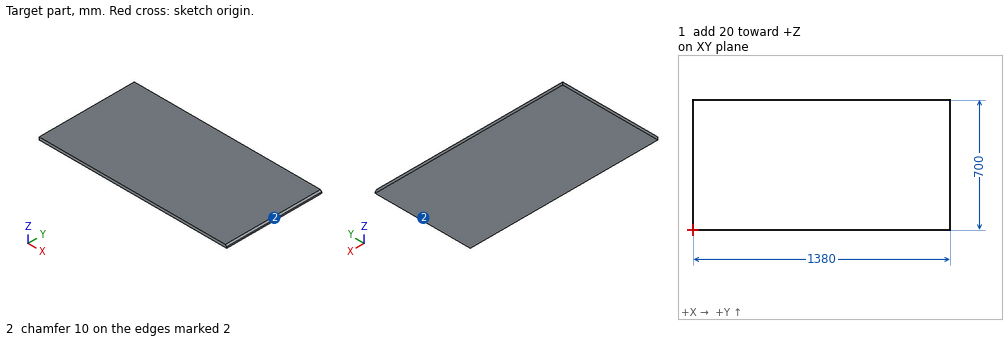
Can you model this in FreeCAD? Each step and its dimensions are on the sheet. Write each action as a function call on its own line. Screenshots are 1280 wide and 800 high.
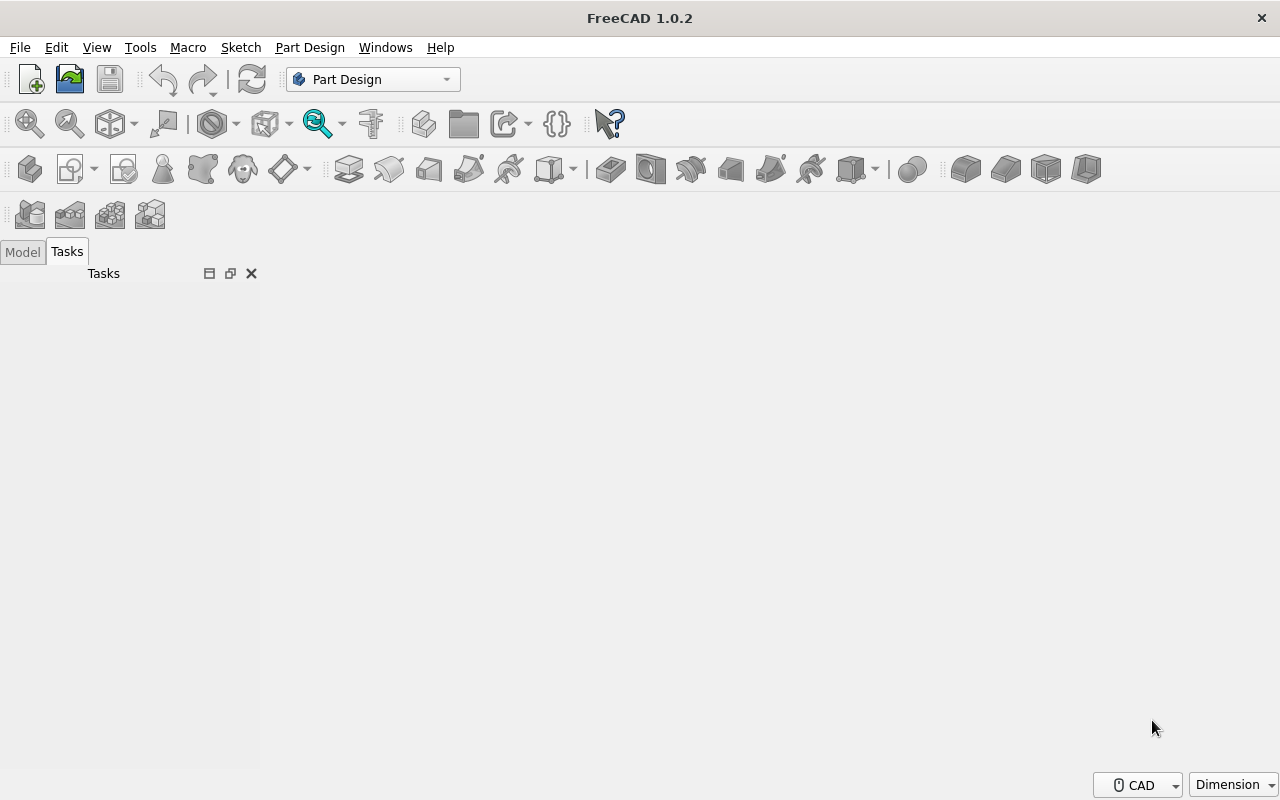
click(30, 80)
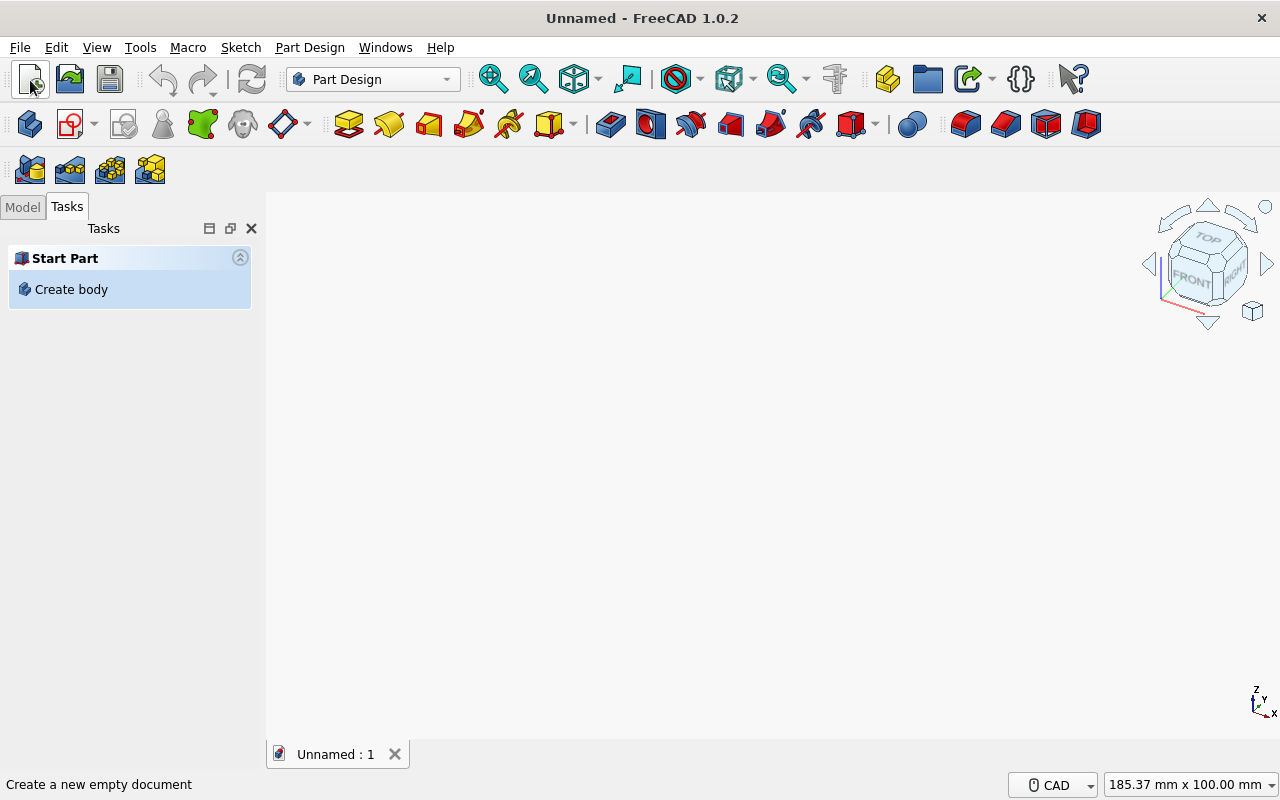
click(70, 124)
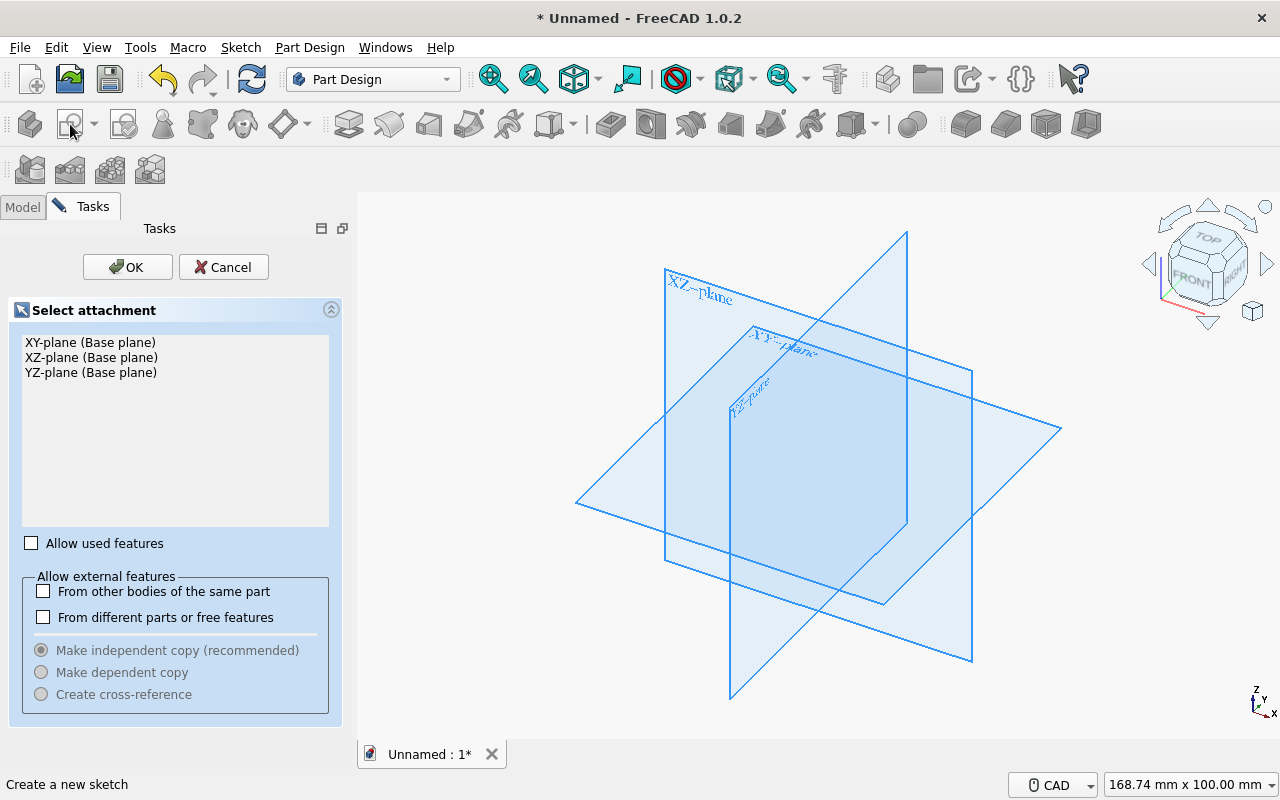
click(82, 342)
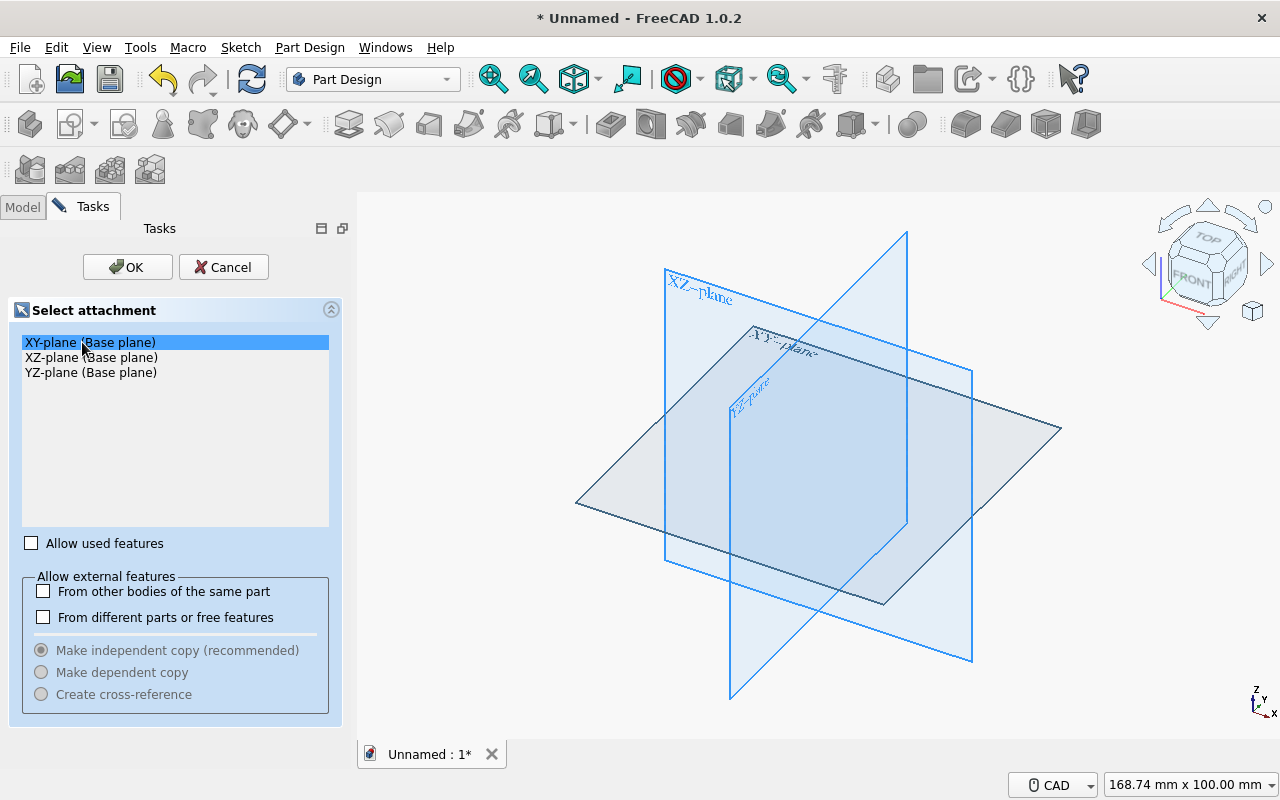
click(128, 267)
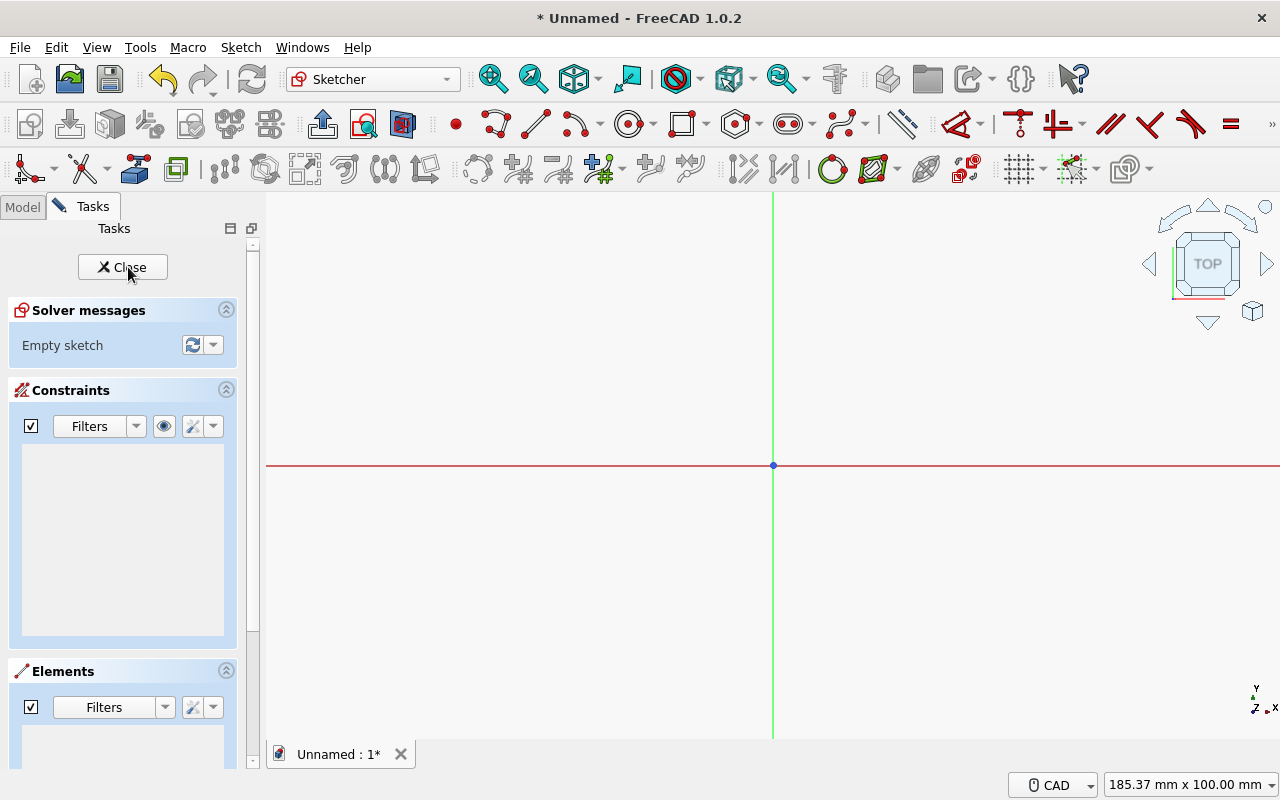
scroll(396, 619, down, 13)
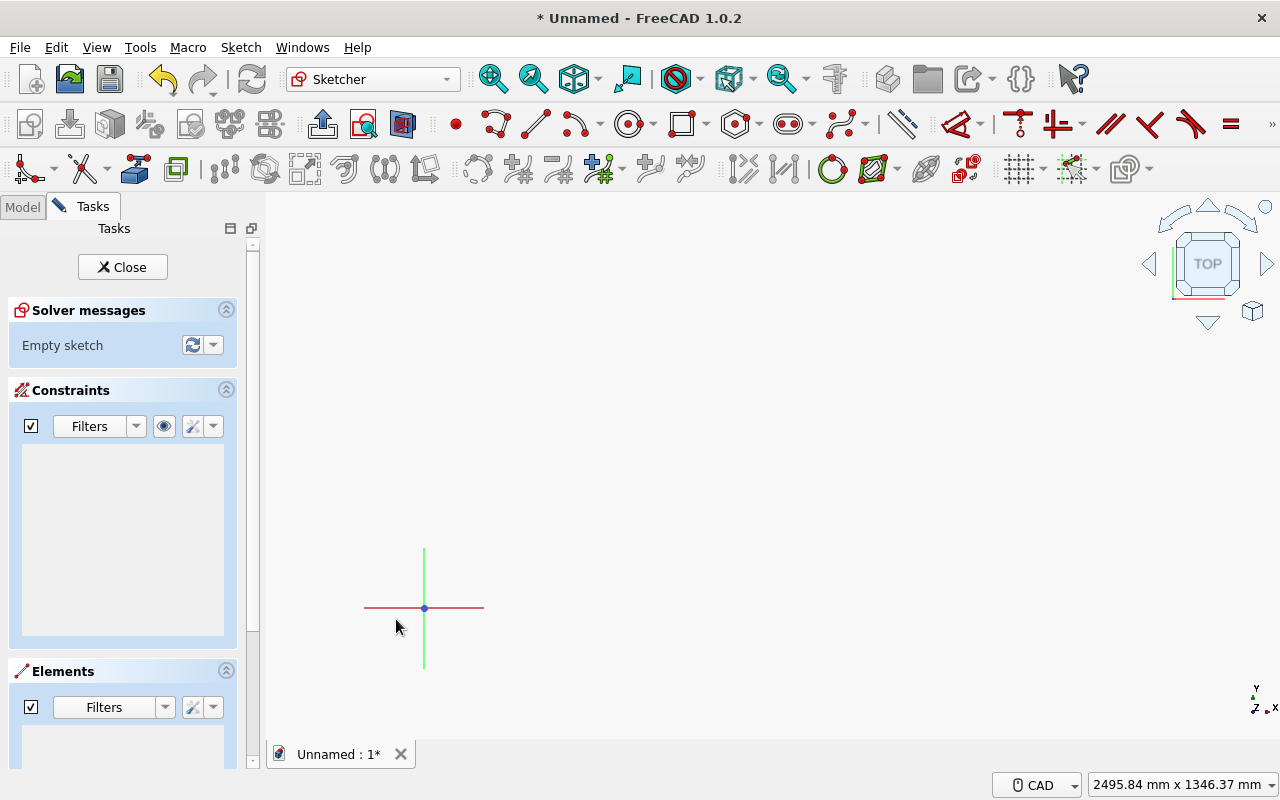
click(682, 124)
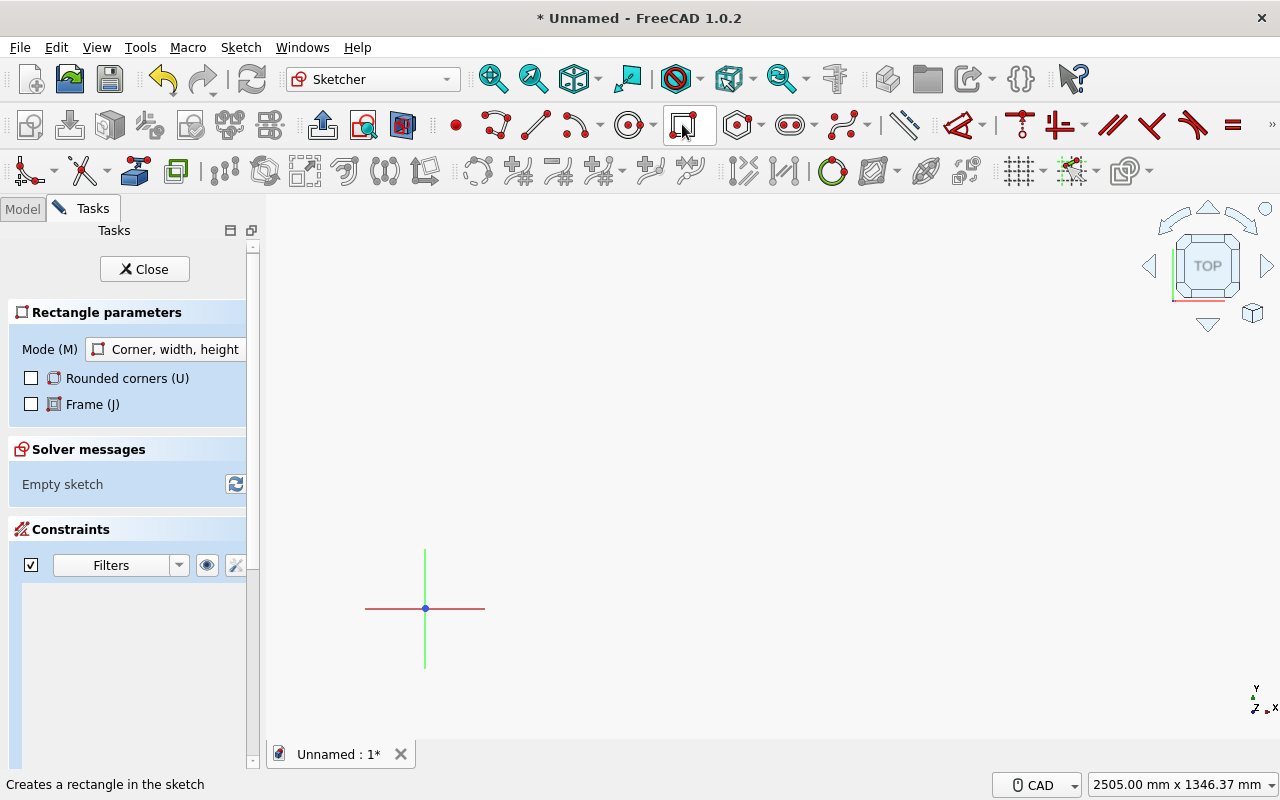
click(425, 609)
move(984, 325)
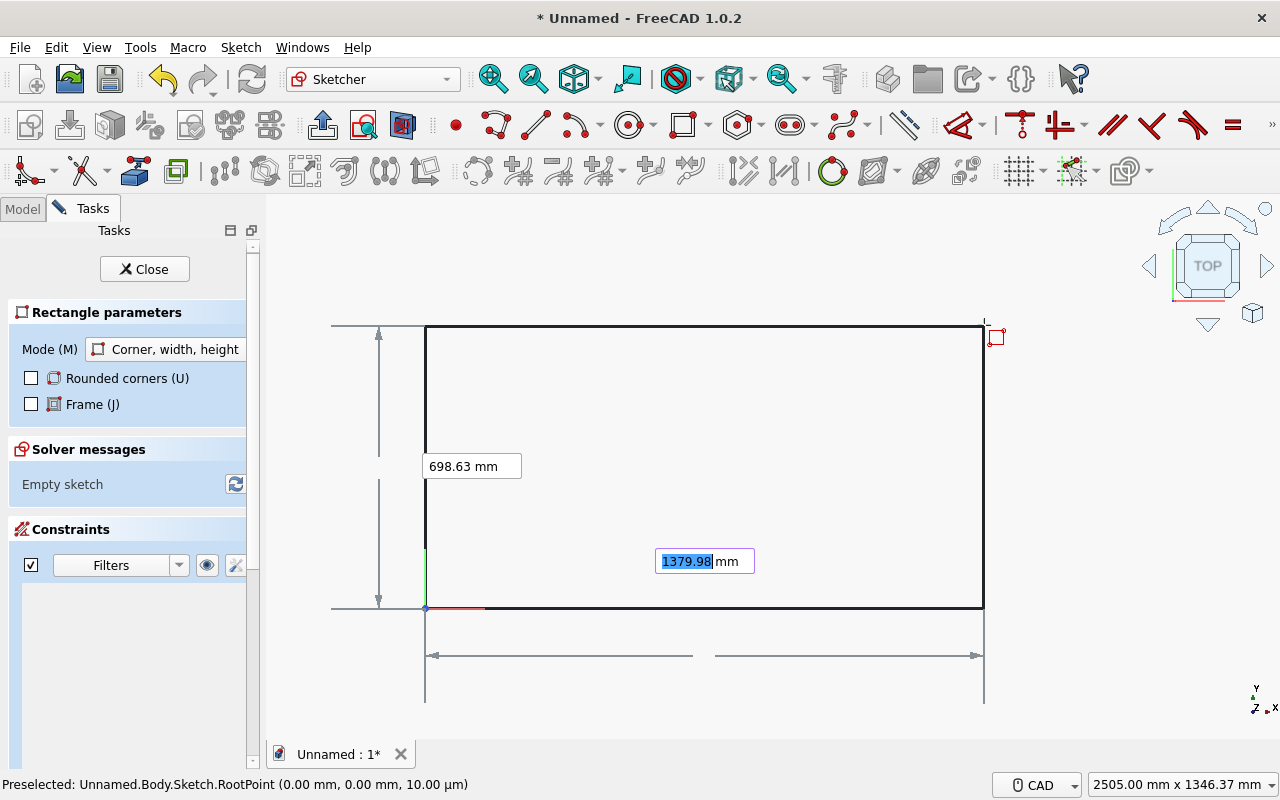
text(1380)
key(Tab)
text(700)
key(Return)
key(Escape)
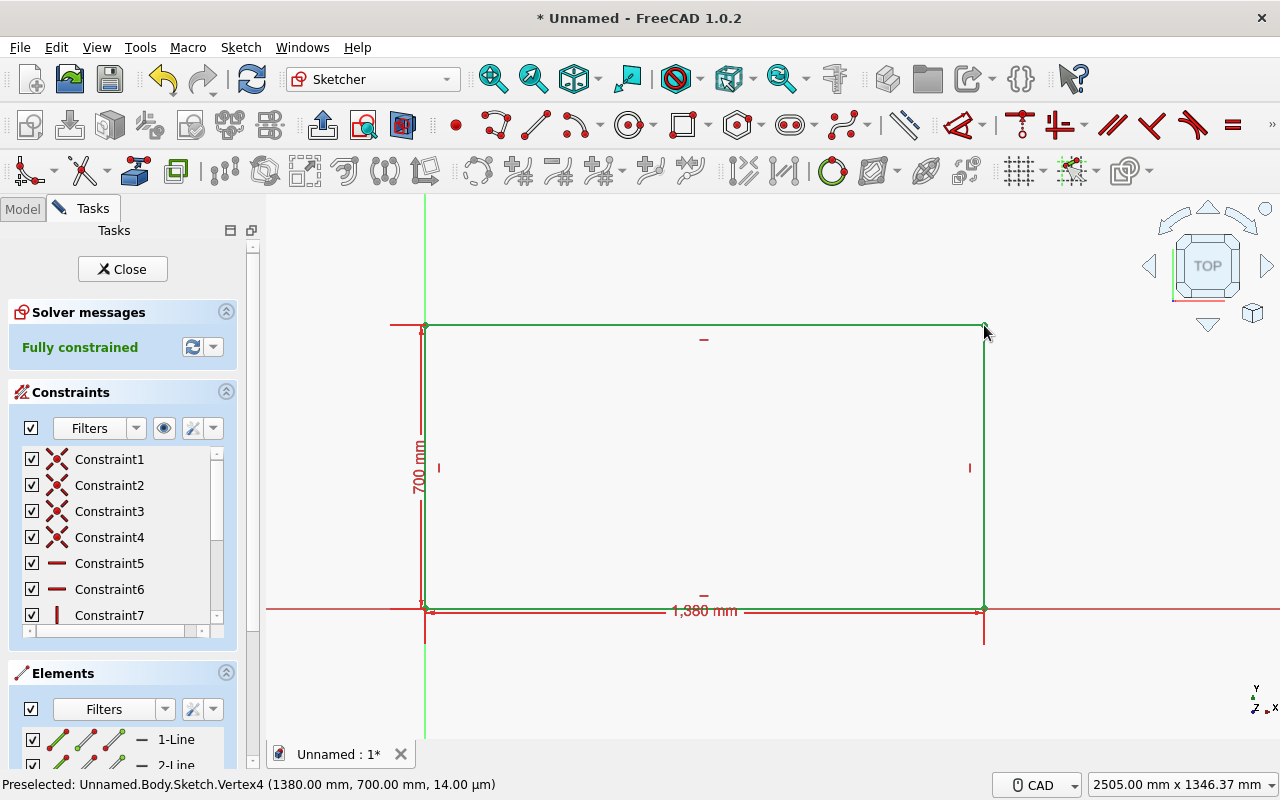
click(123, 269)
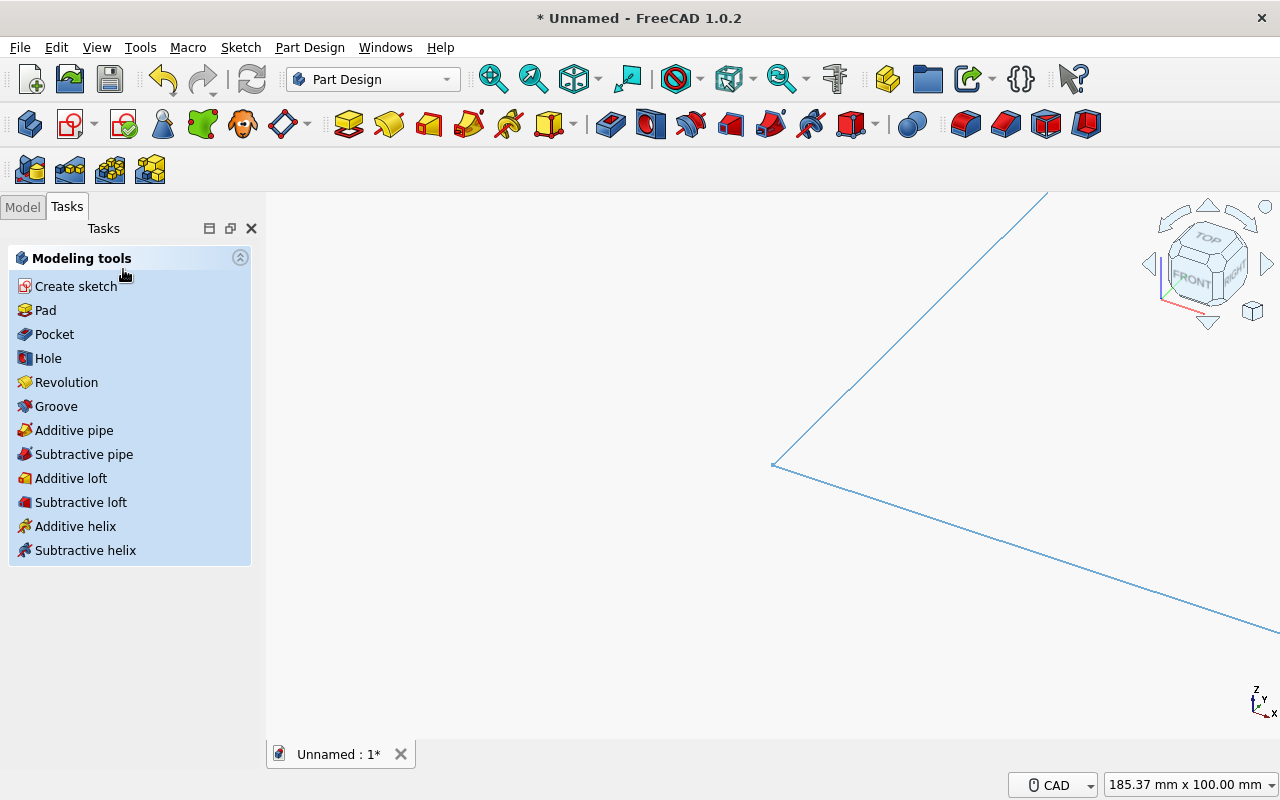
click(350, 124)